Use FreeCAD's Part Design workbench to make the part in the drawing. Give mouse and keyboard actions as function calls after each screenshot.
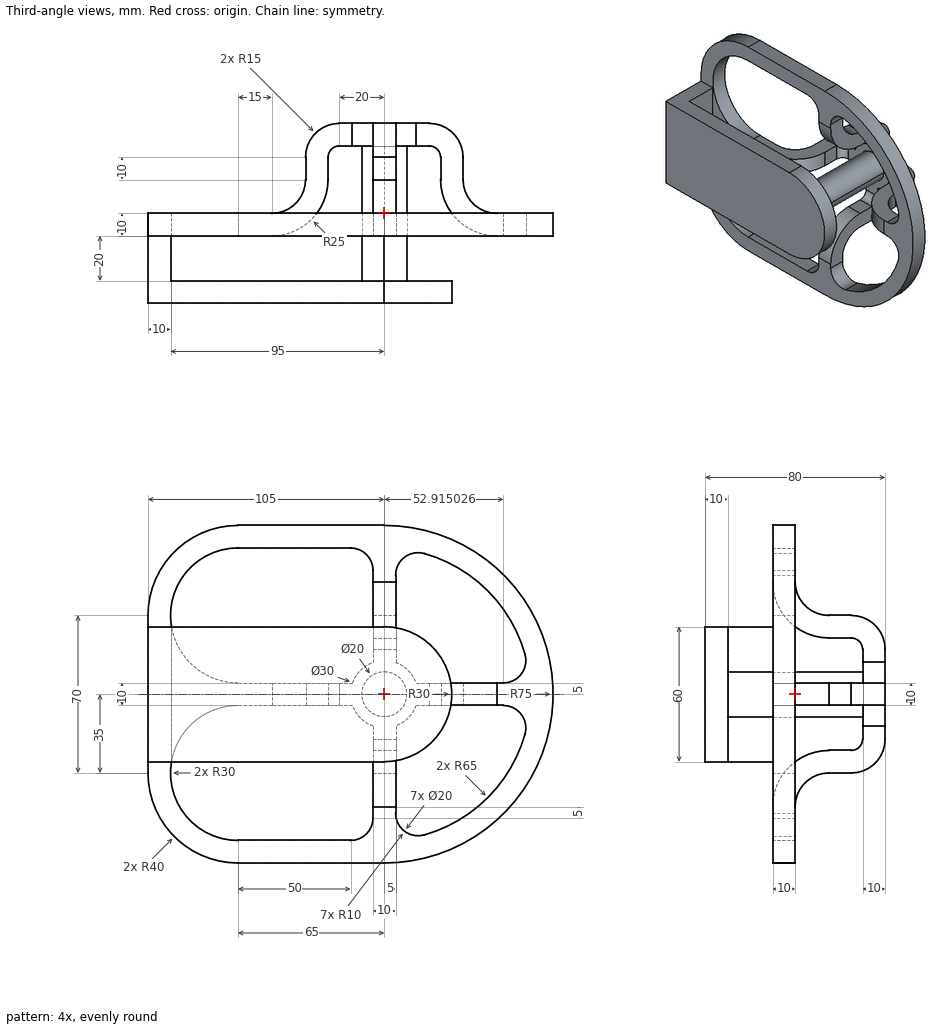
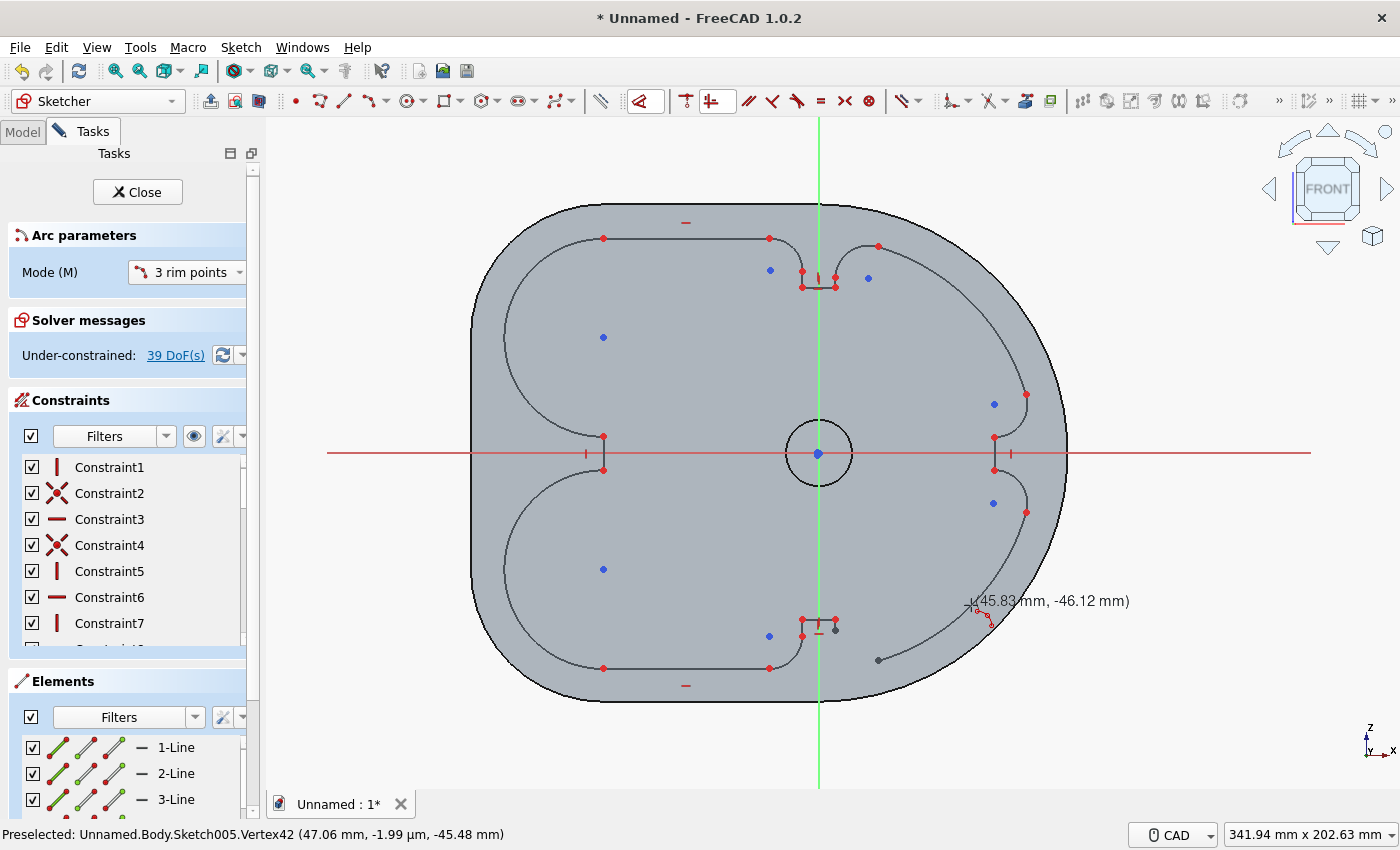
click(878, 661)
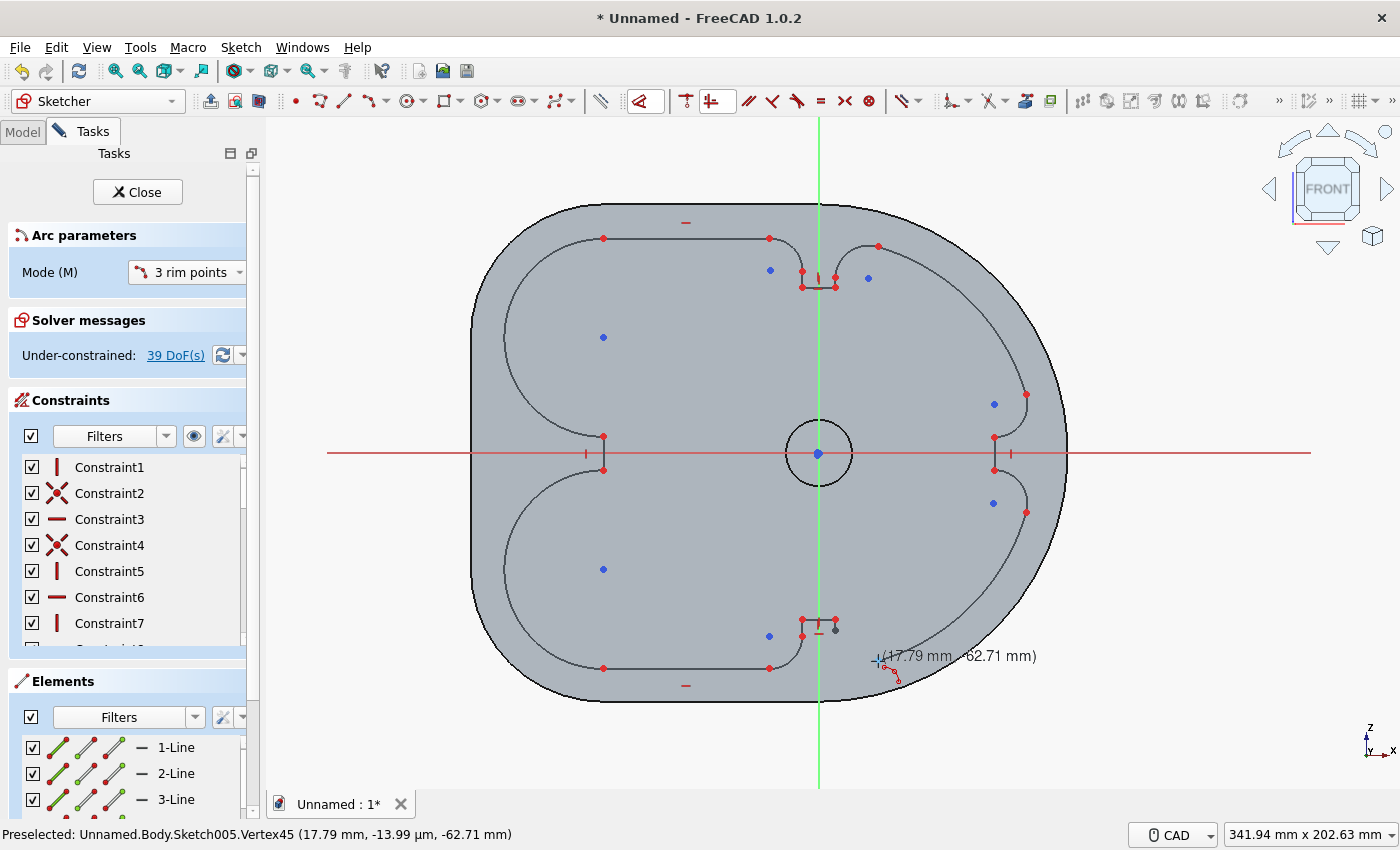
scroll(836, 629, up, 6)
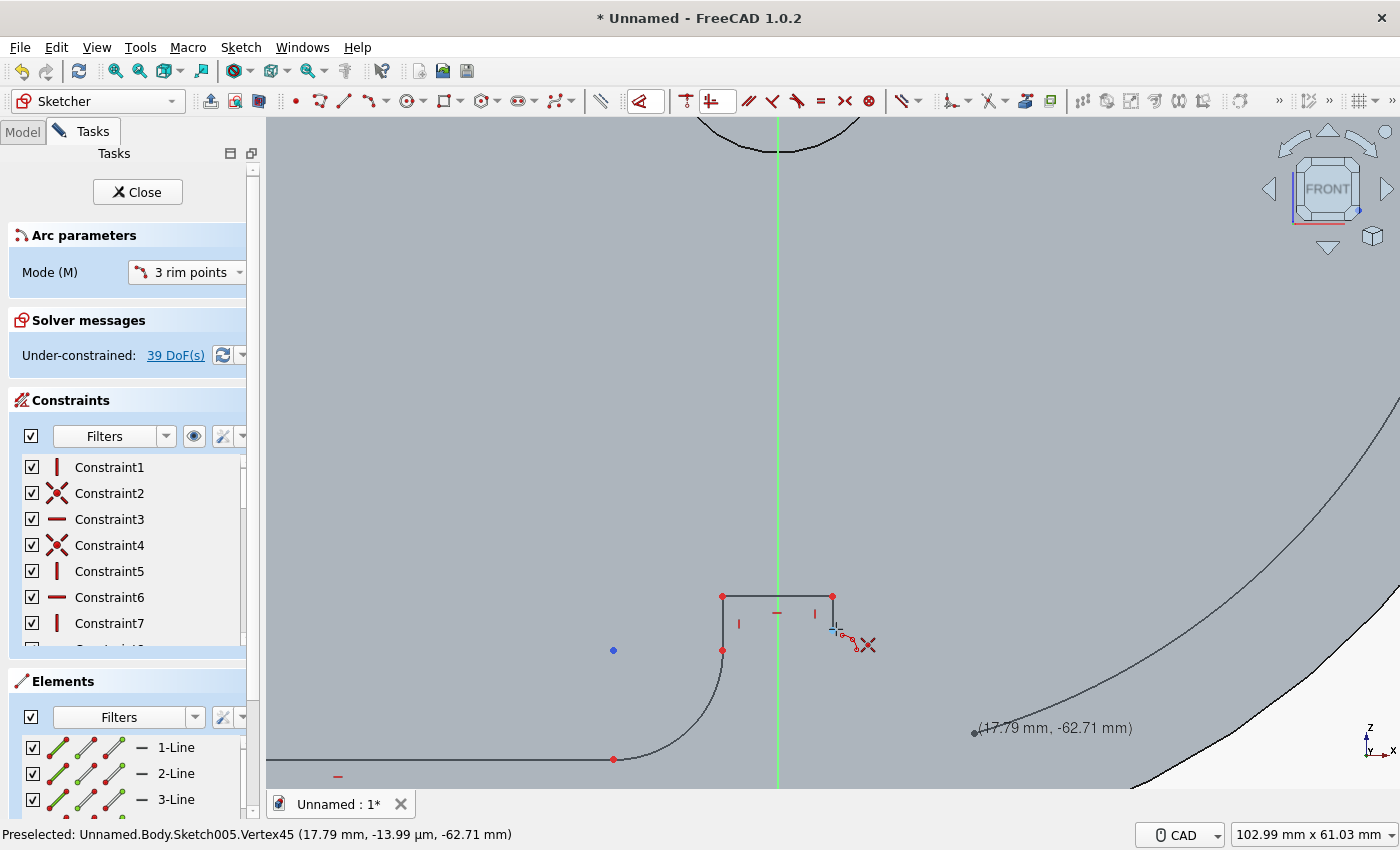
click(833, 631)
click(877, 714)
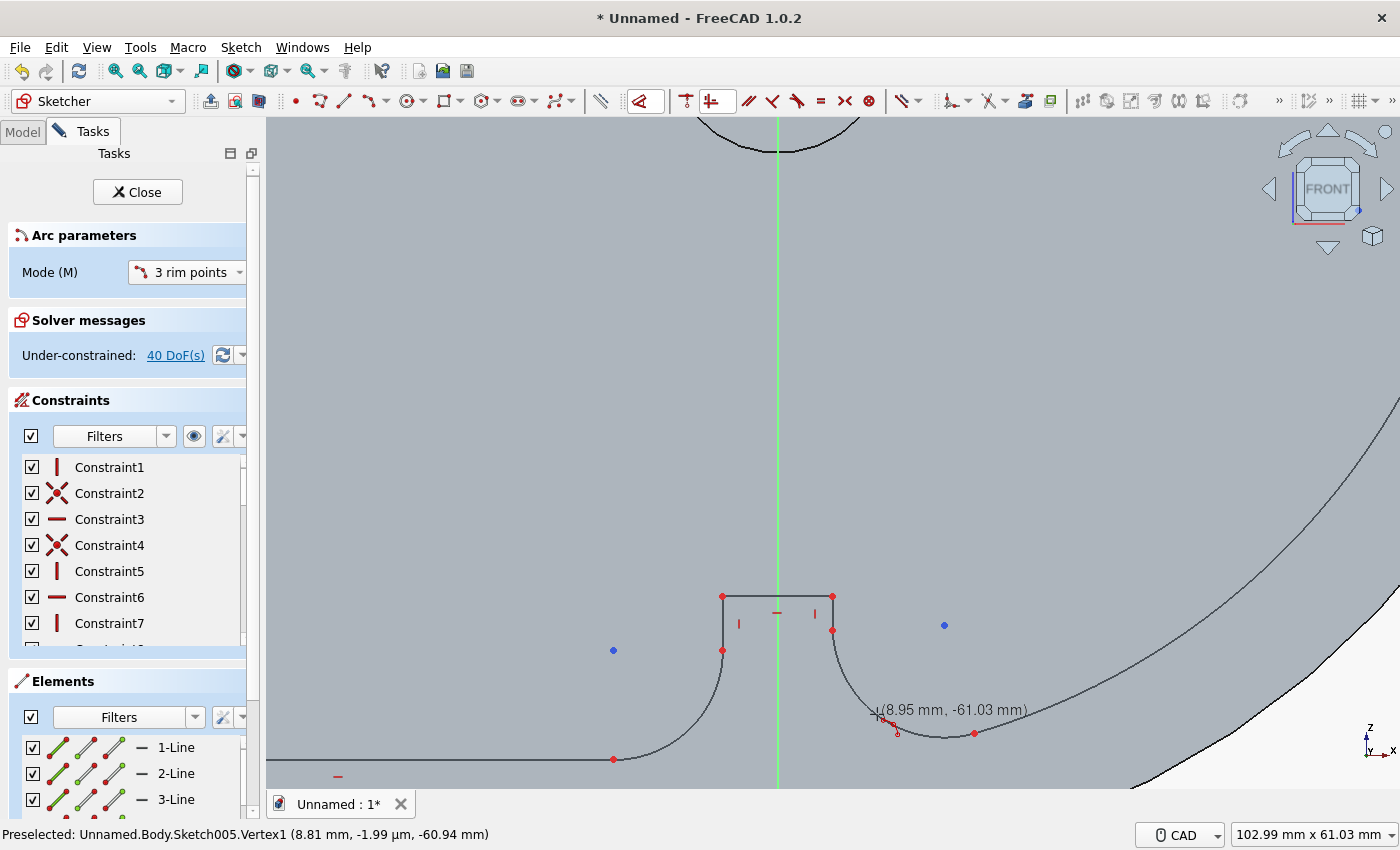
click(408, 102)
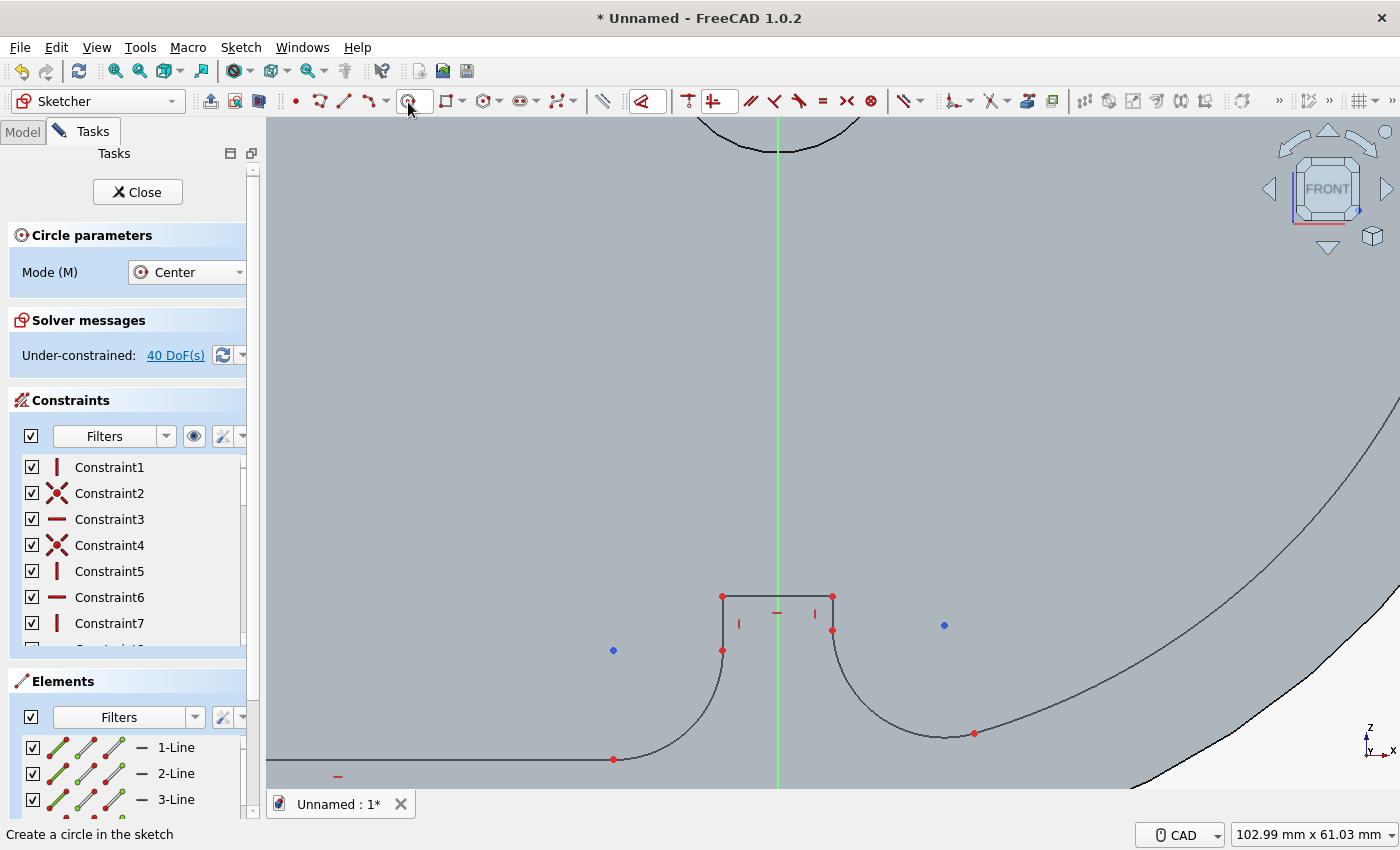
scroll(836, 630, down, 6)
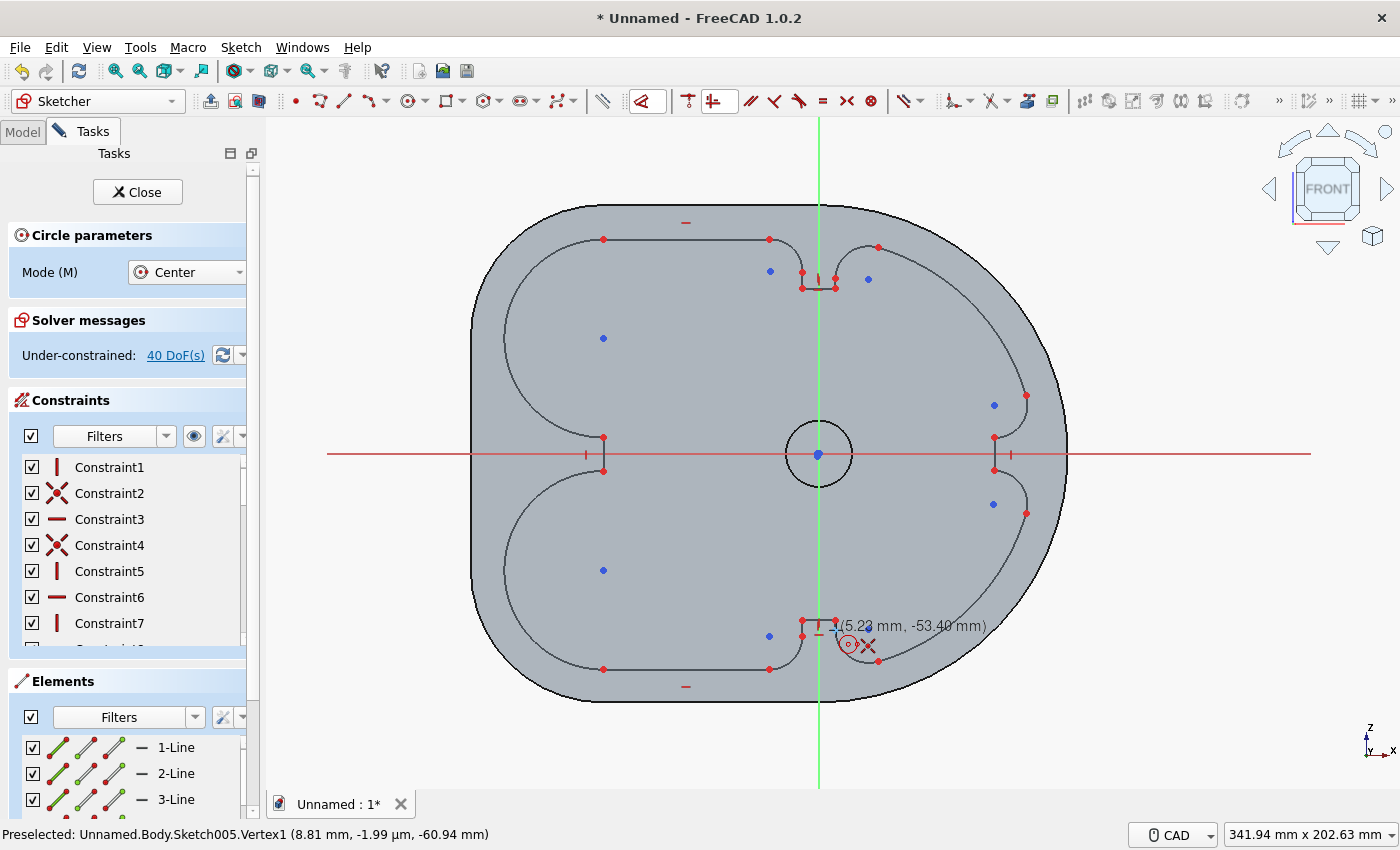
click(819, 454)
move(842, 430)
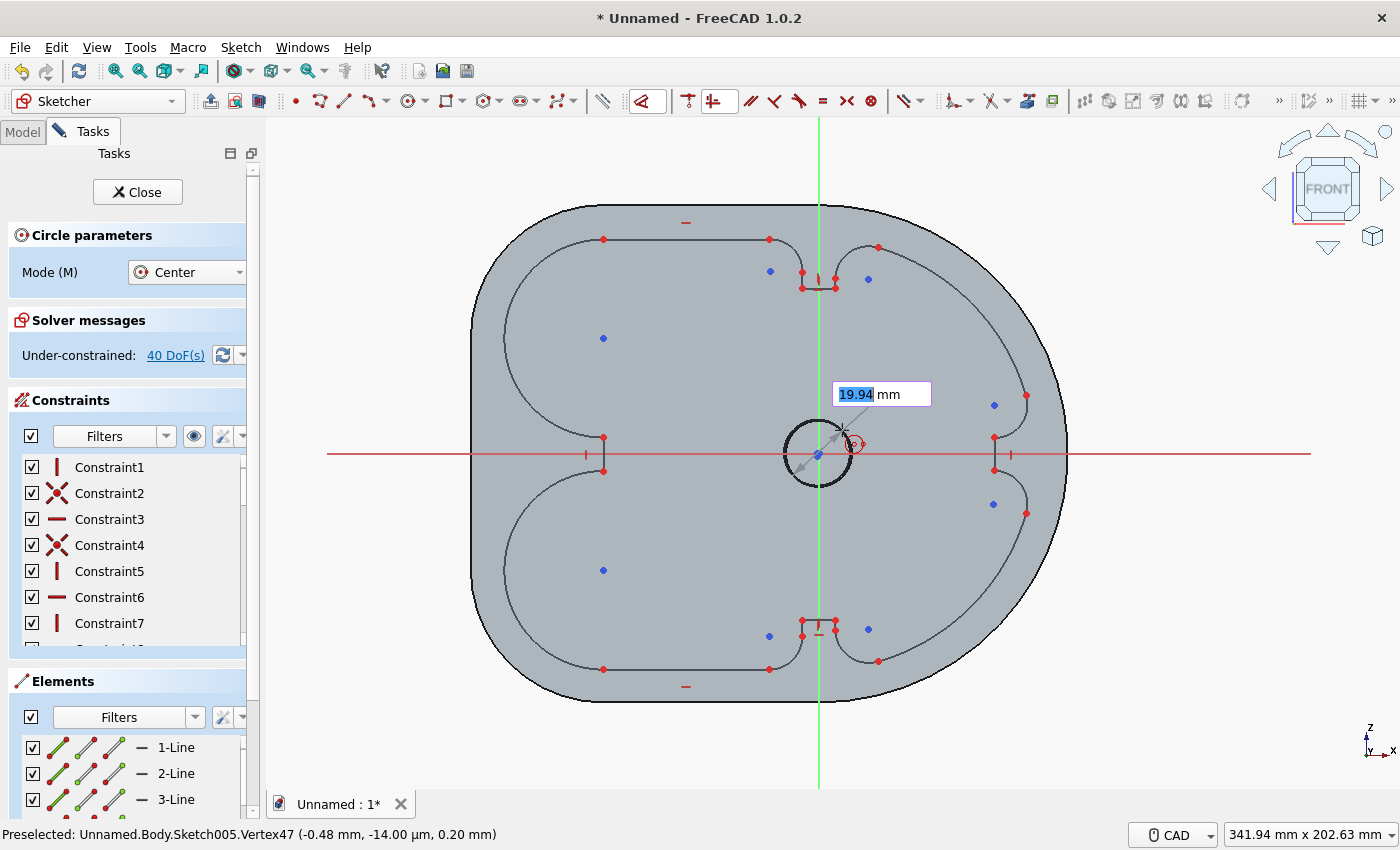
text(20)
key(Return)
key(Escape)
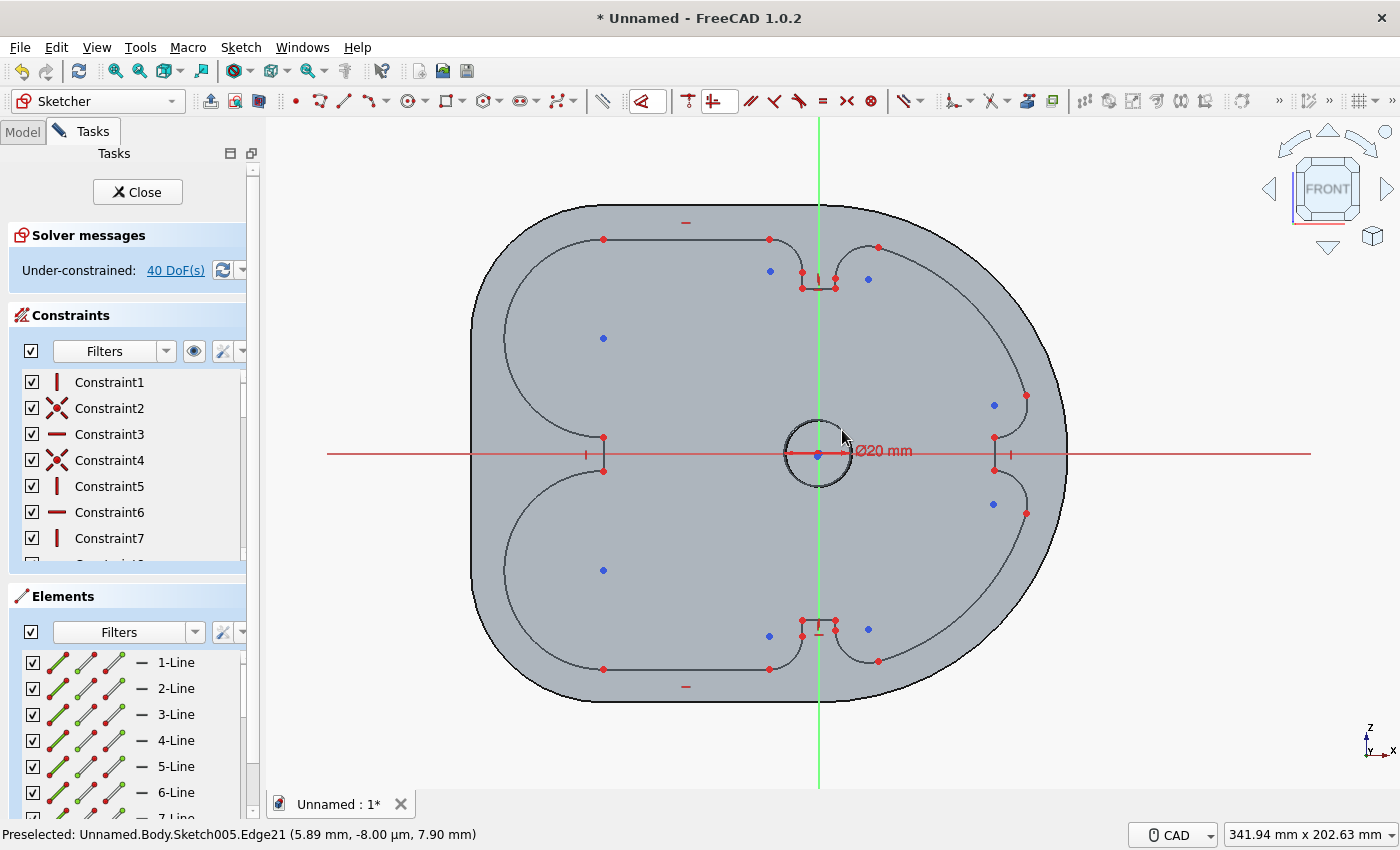
scroll(835, 626, up, 5)